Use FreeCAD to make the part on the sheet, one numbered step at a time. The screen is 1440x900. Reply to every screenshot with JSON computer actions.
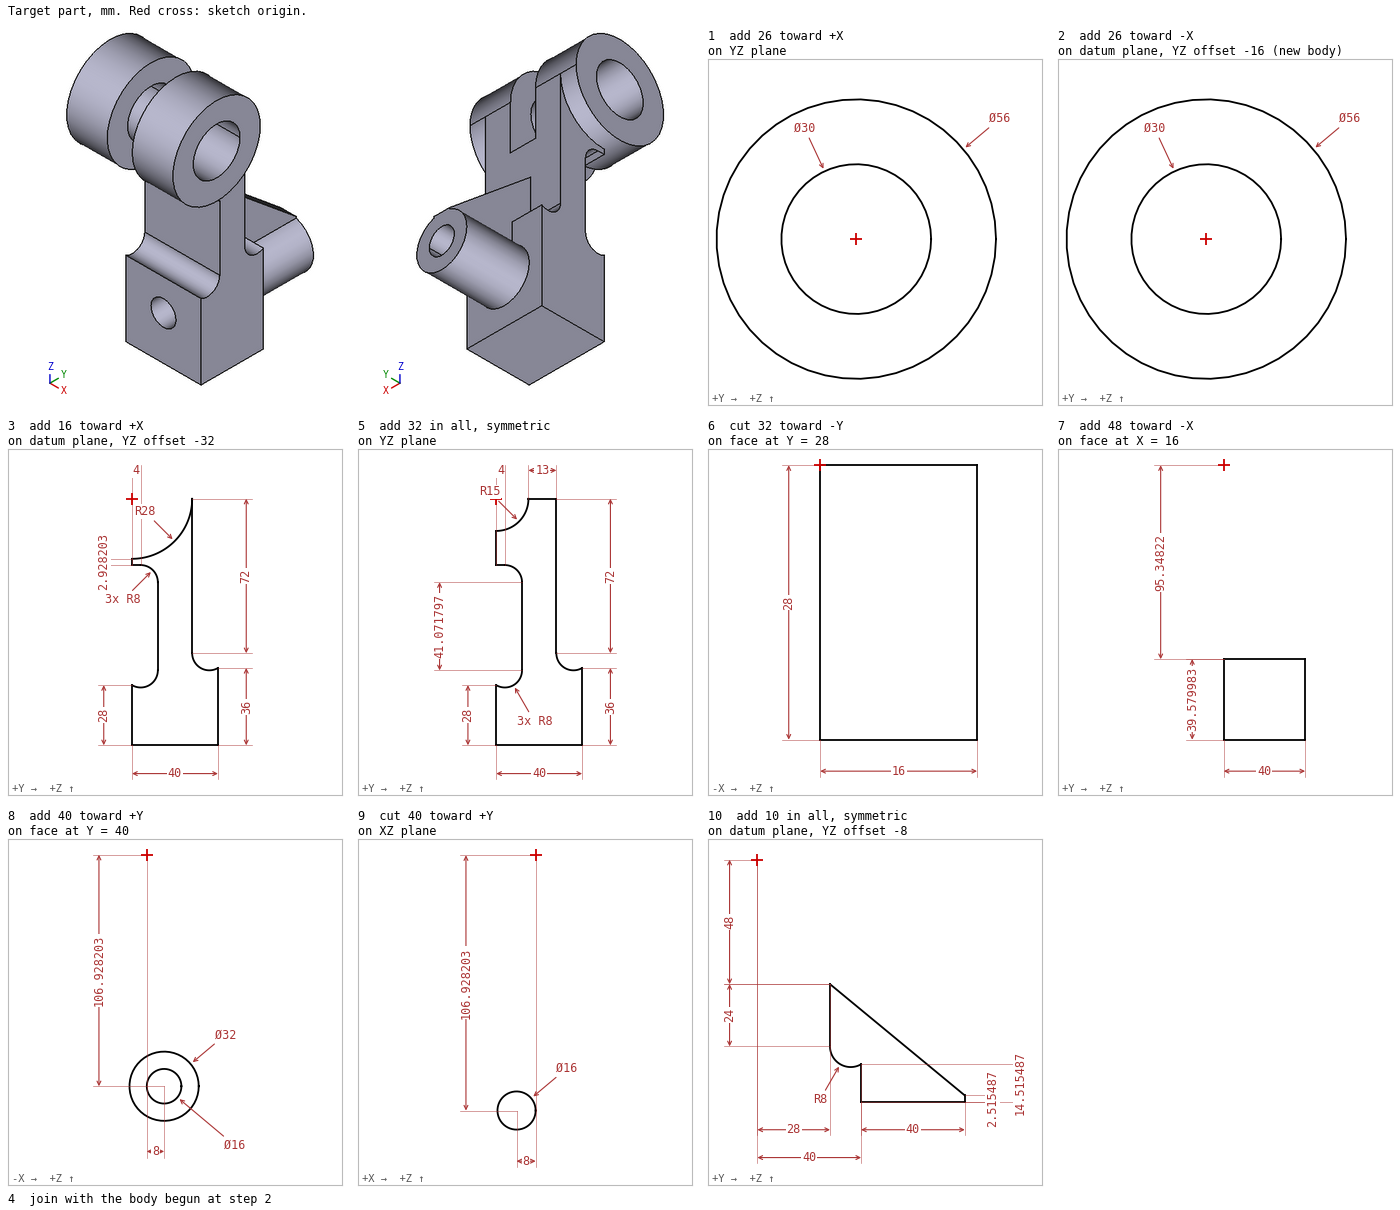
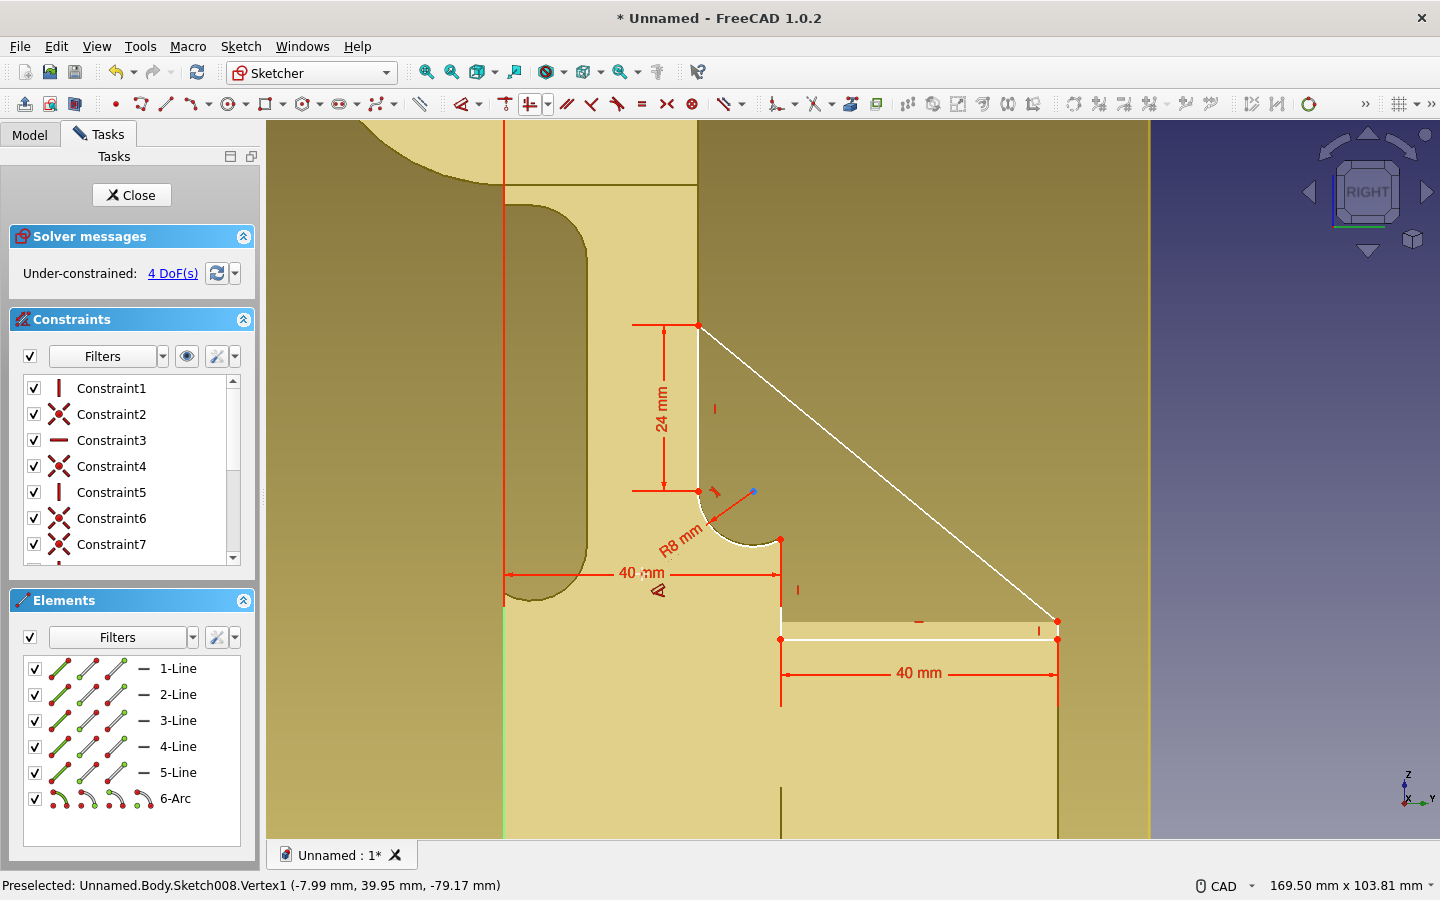
{"action": "left_click", "coordinate": [698, 325]}
{"action": "left_click", "coordinate": [601, 359]}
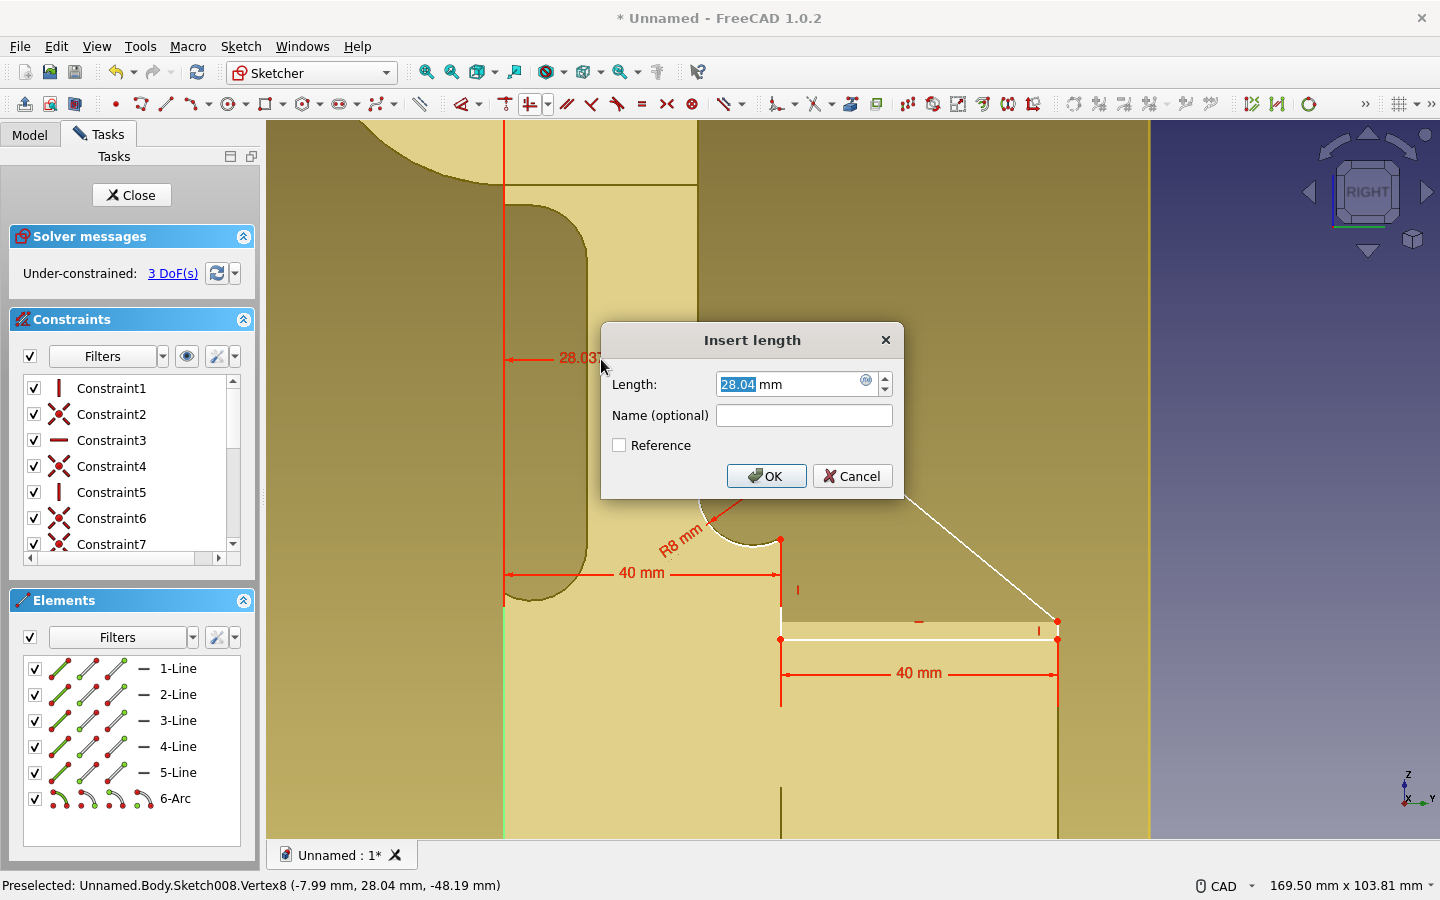
{"action": "type", "text": "28"}
{"action": "key", "text": "Return"}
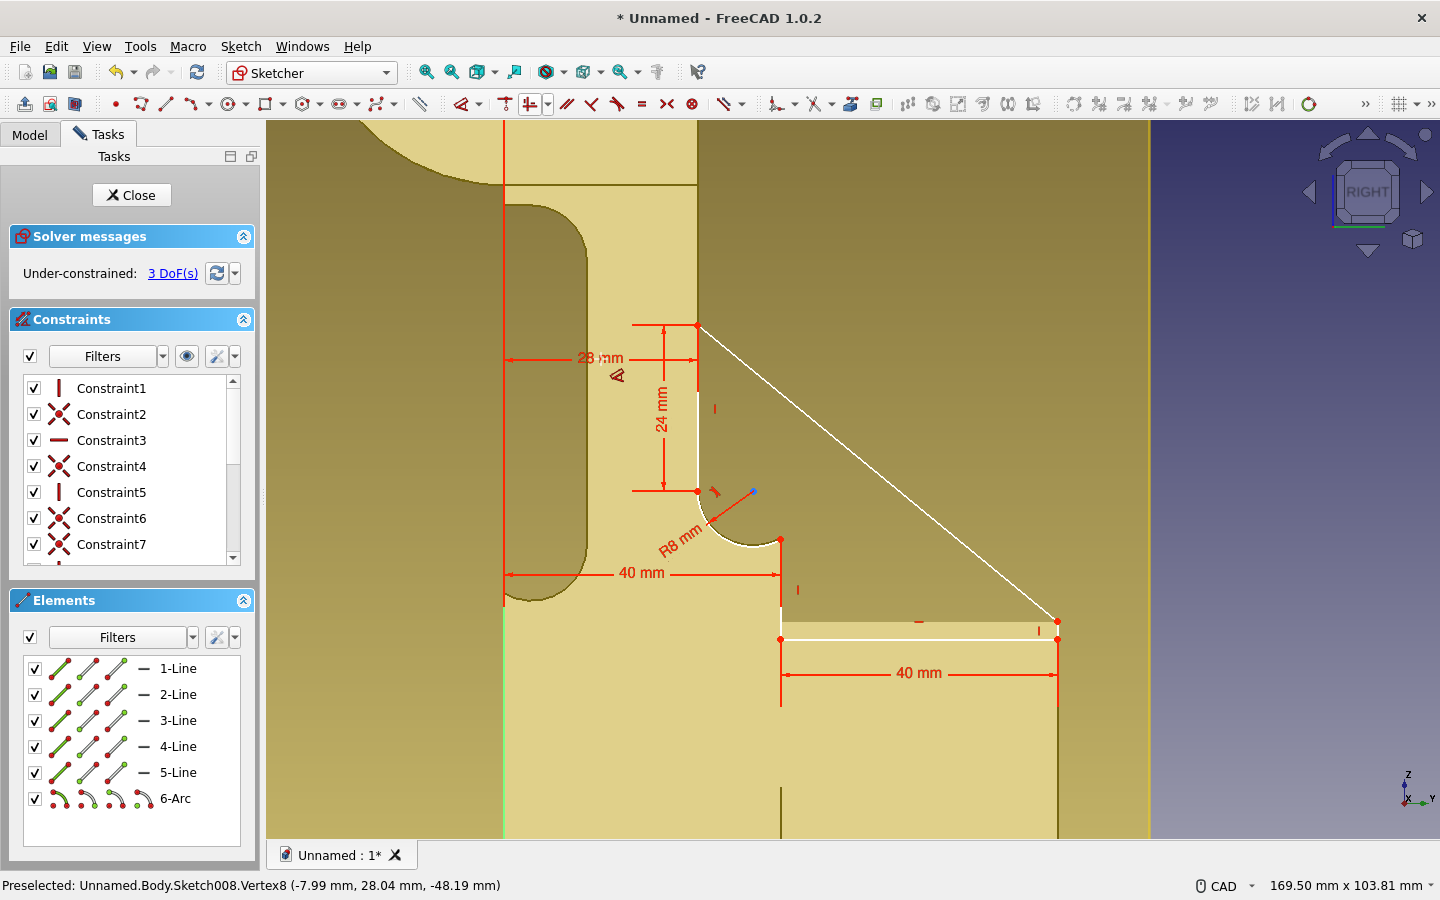
{"action": "left_click", "coordinate": [698, 325]}
{"action": "left_click", "coordinate": [470, 237]}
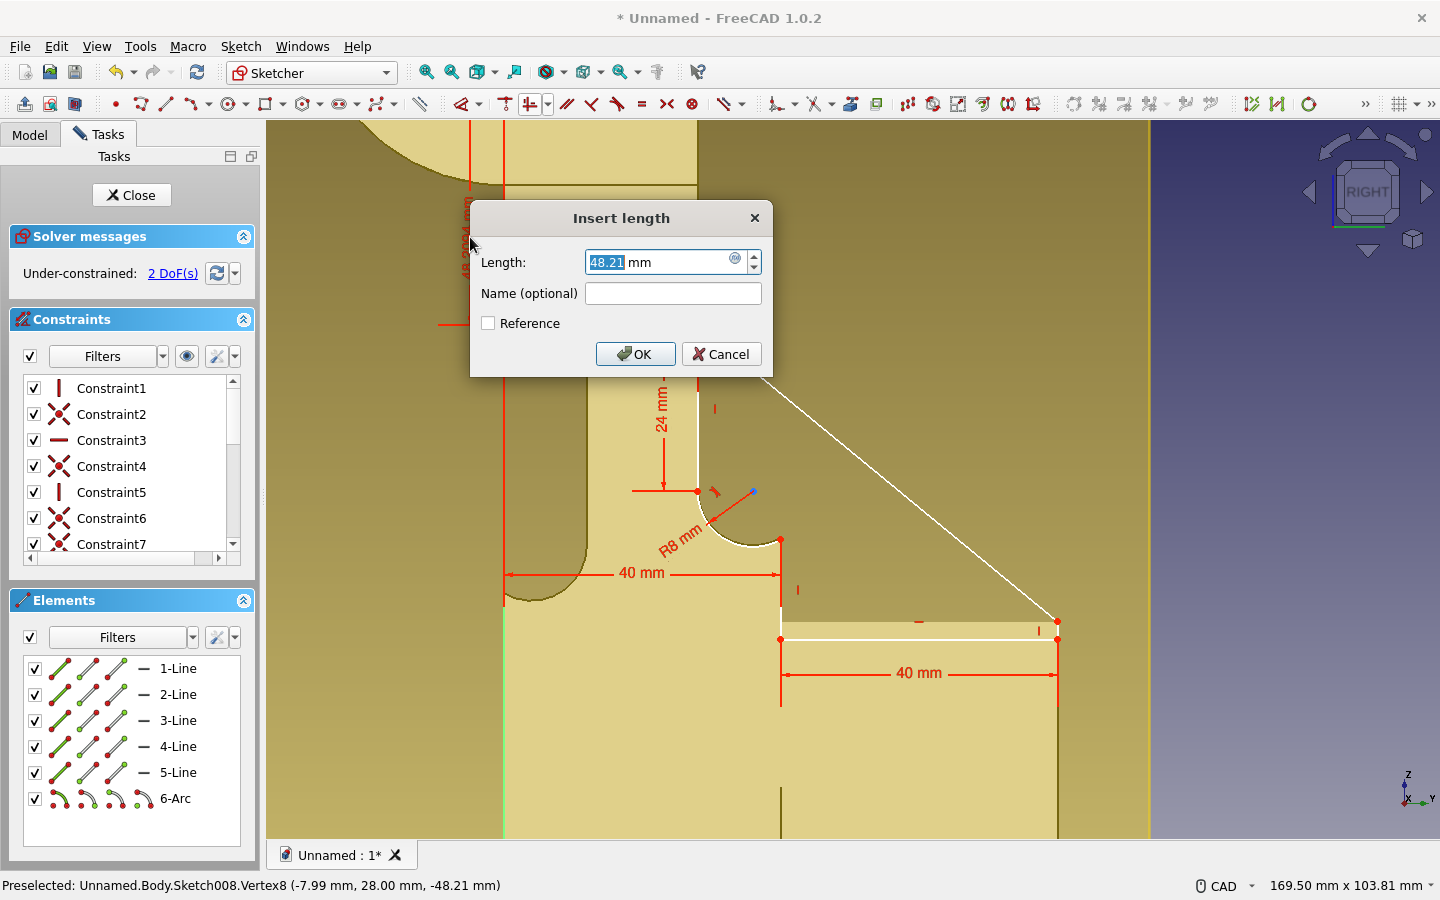
{"action": "type", "text": "48"}
{"action": "key", "text": "Return"}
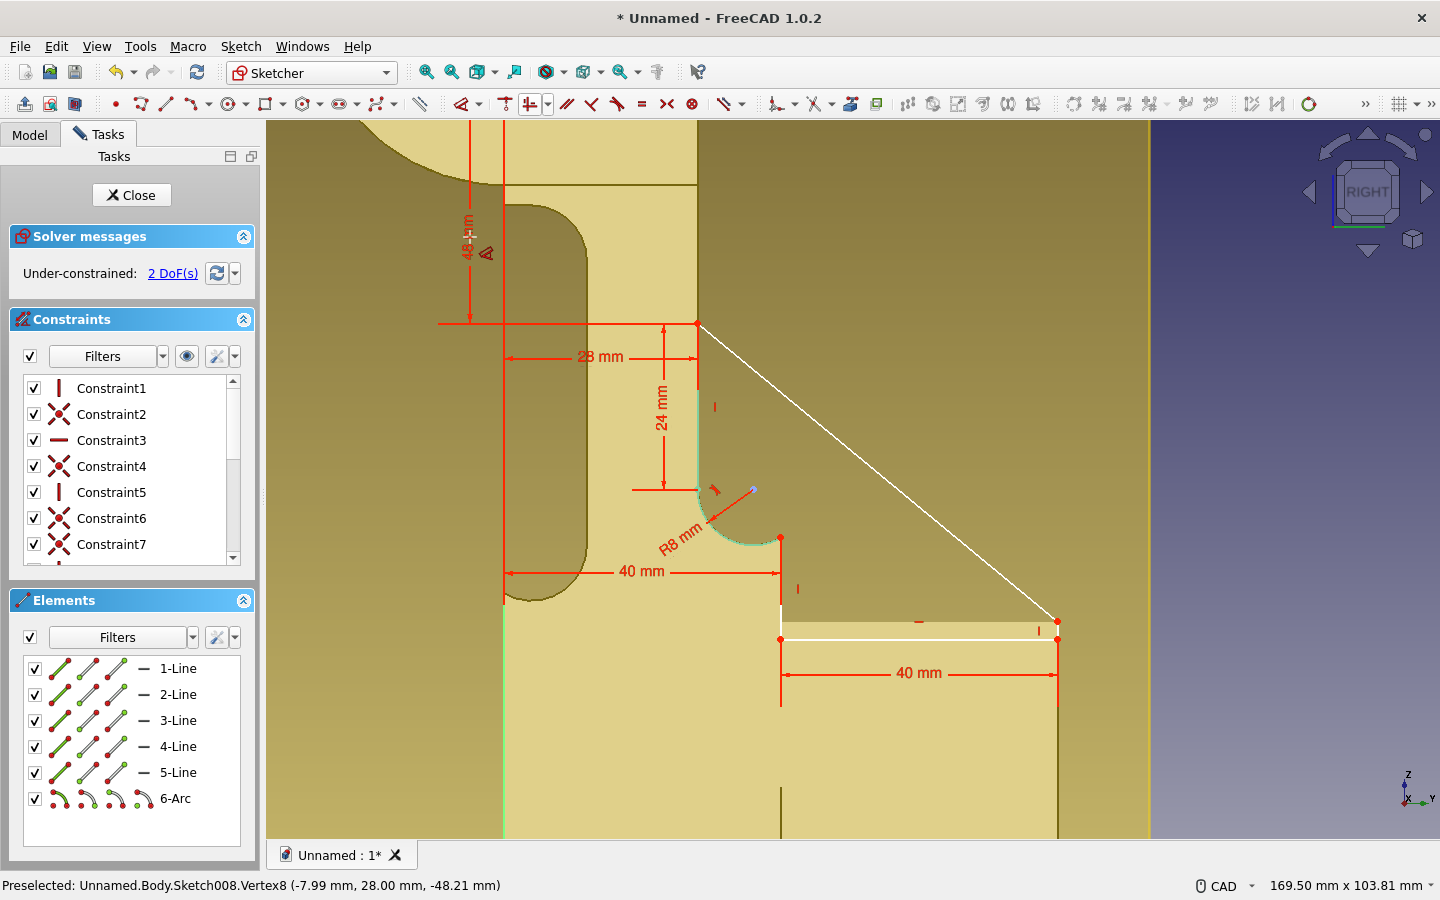
{"action": "scroll", "coordinate": [1058, 631], "scroll_direction": "up", "scroll_amount": 5}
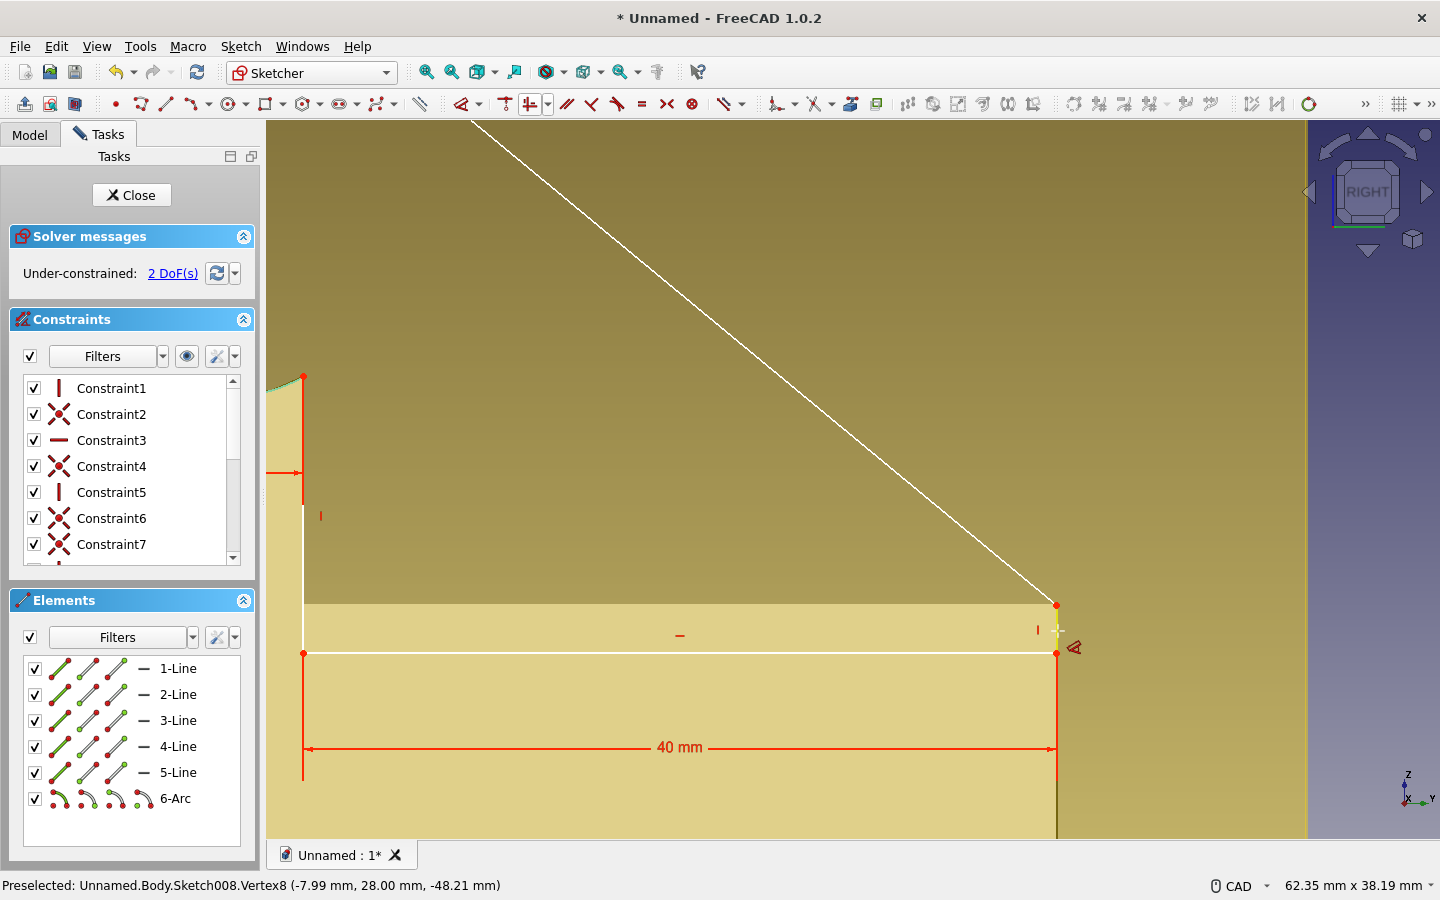
{"action": "left_click", "coordinate": [1057, 629]}
{"action": "left_click", "coordinate": [1091, 629]}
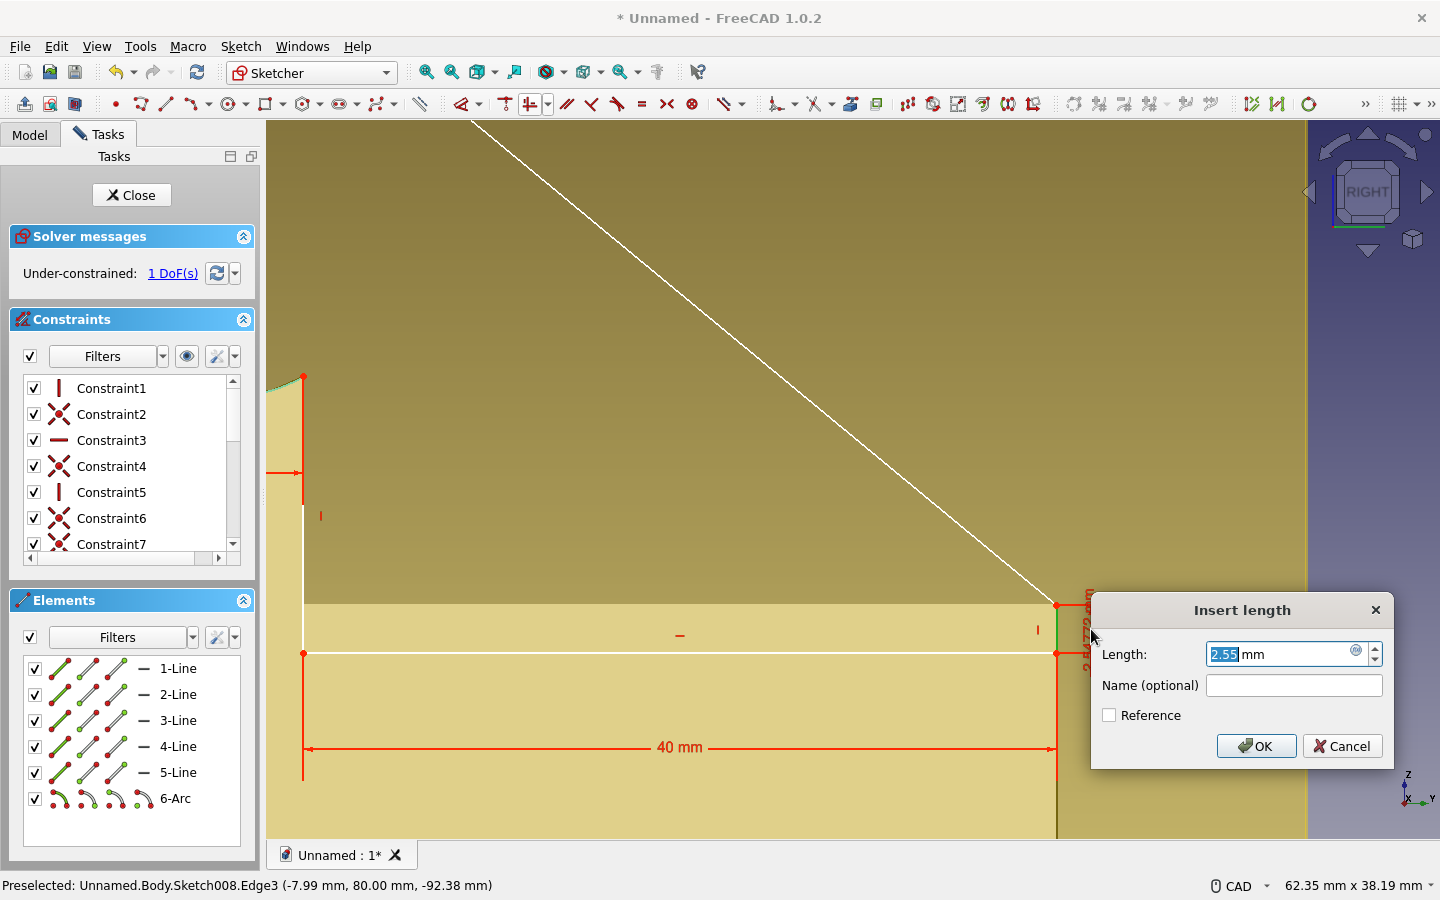
{"action": "type", "text": "2.515487"}
{"action": "key", "text": "Return"}